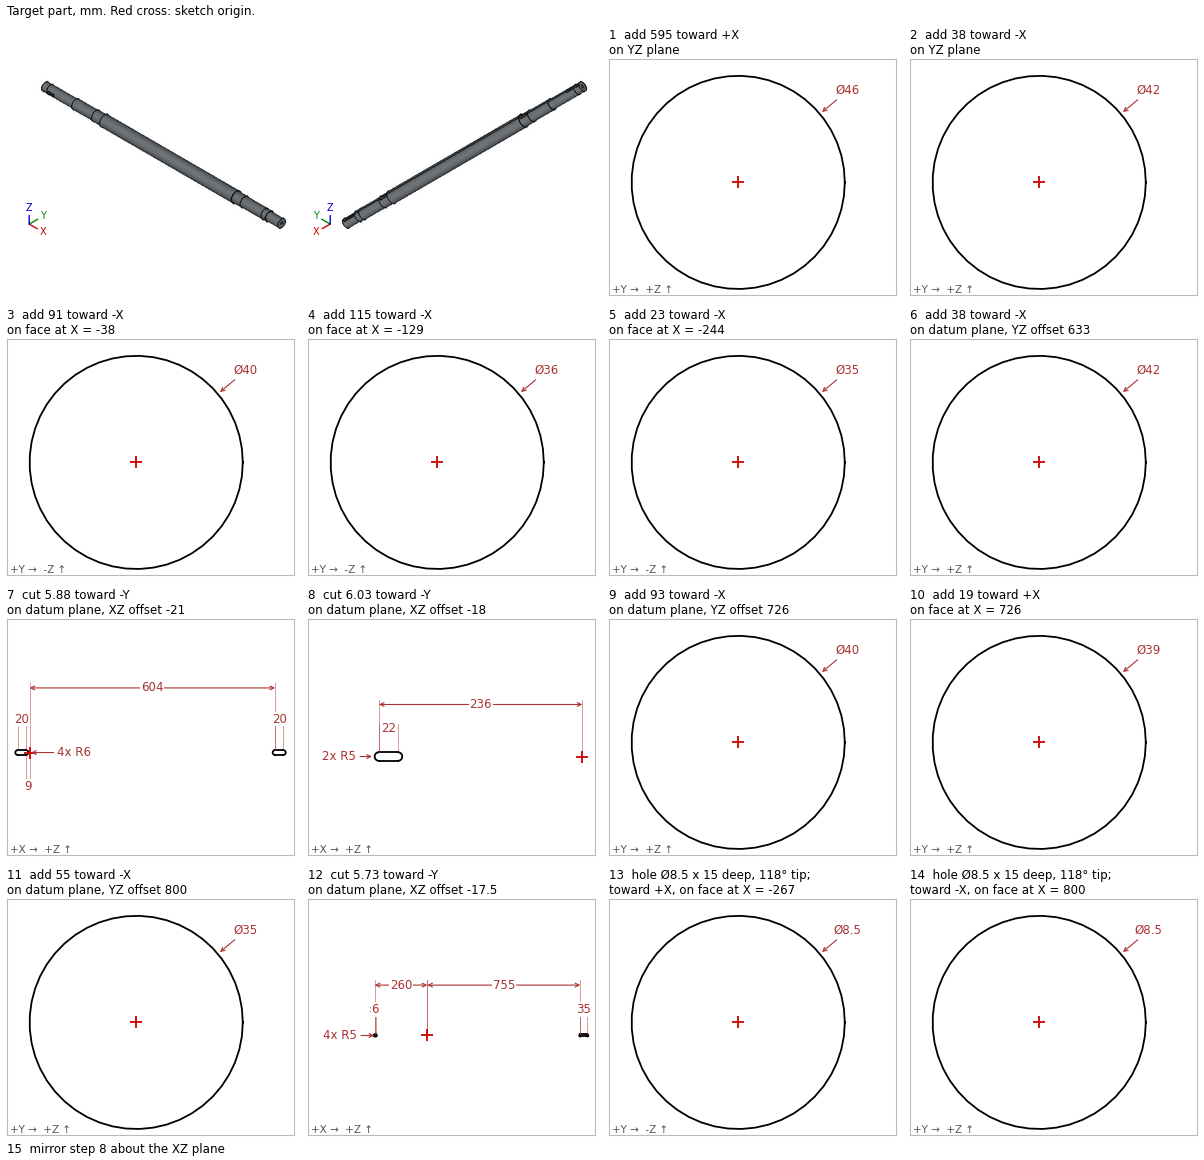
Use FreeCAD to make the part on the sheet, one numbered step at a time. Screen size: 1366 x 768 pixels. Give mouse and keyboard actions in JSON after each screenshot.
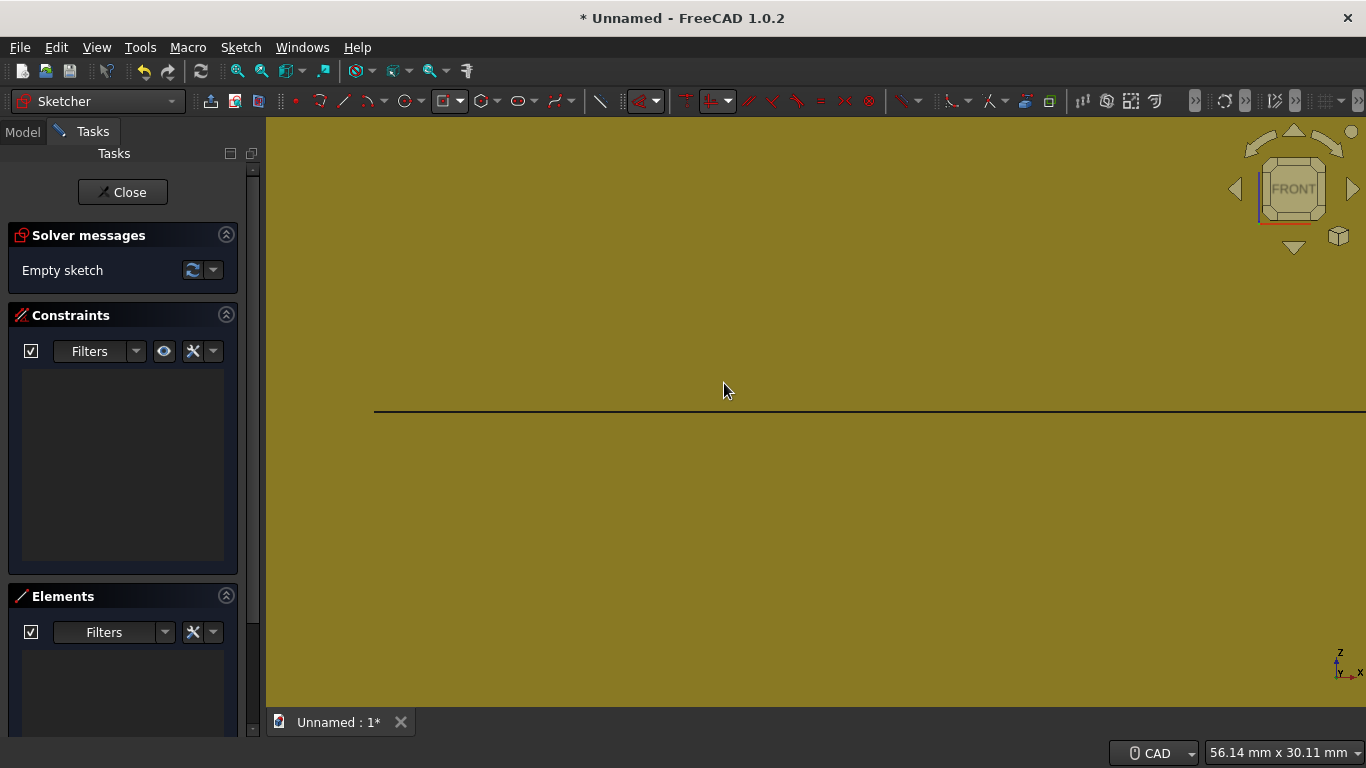
{"action": "key", "text": "g s"}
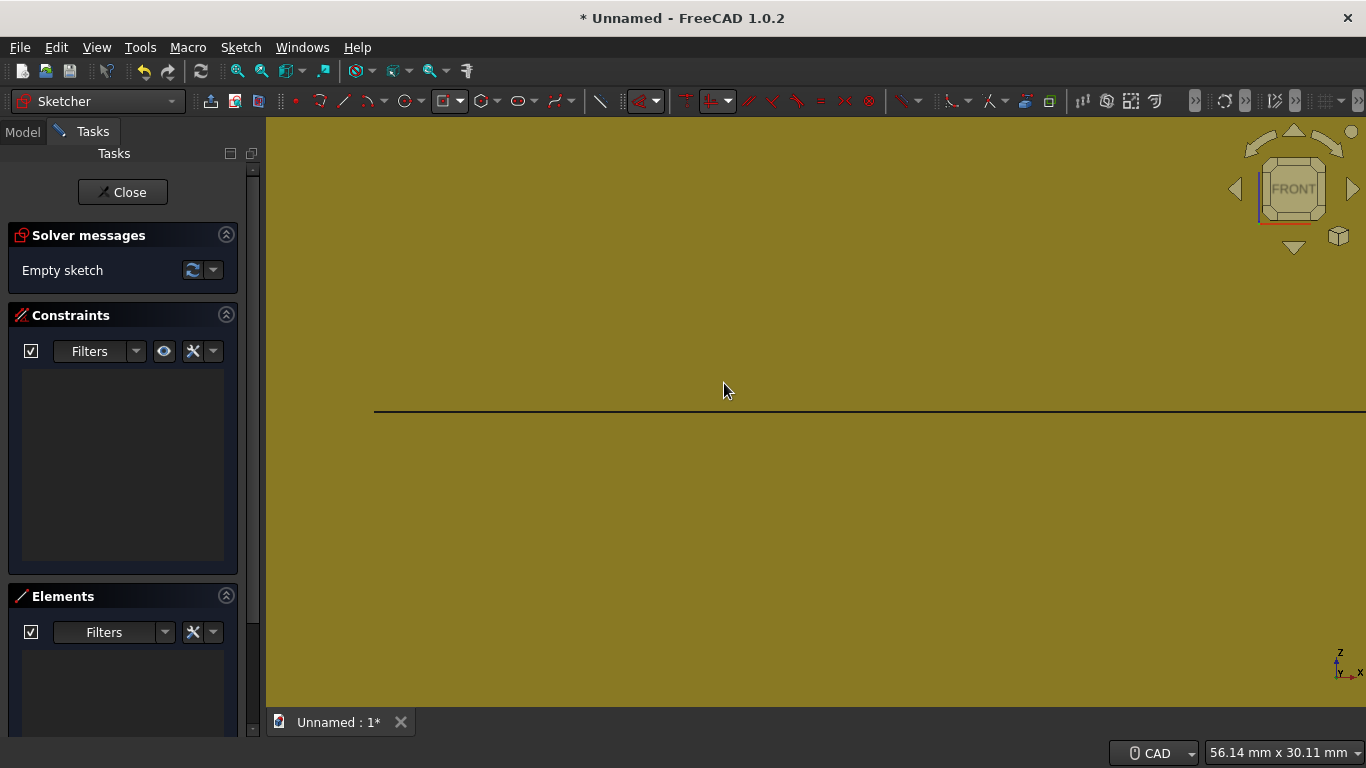
{"action": "left_click", "coordinate": [532, 412]}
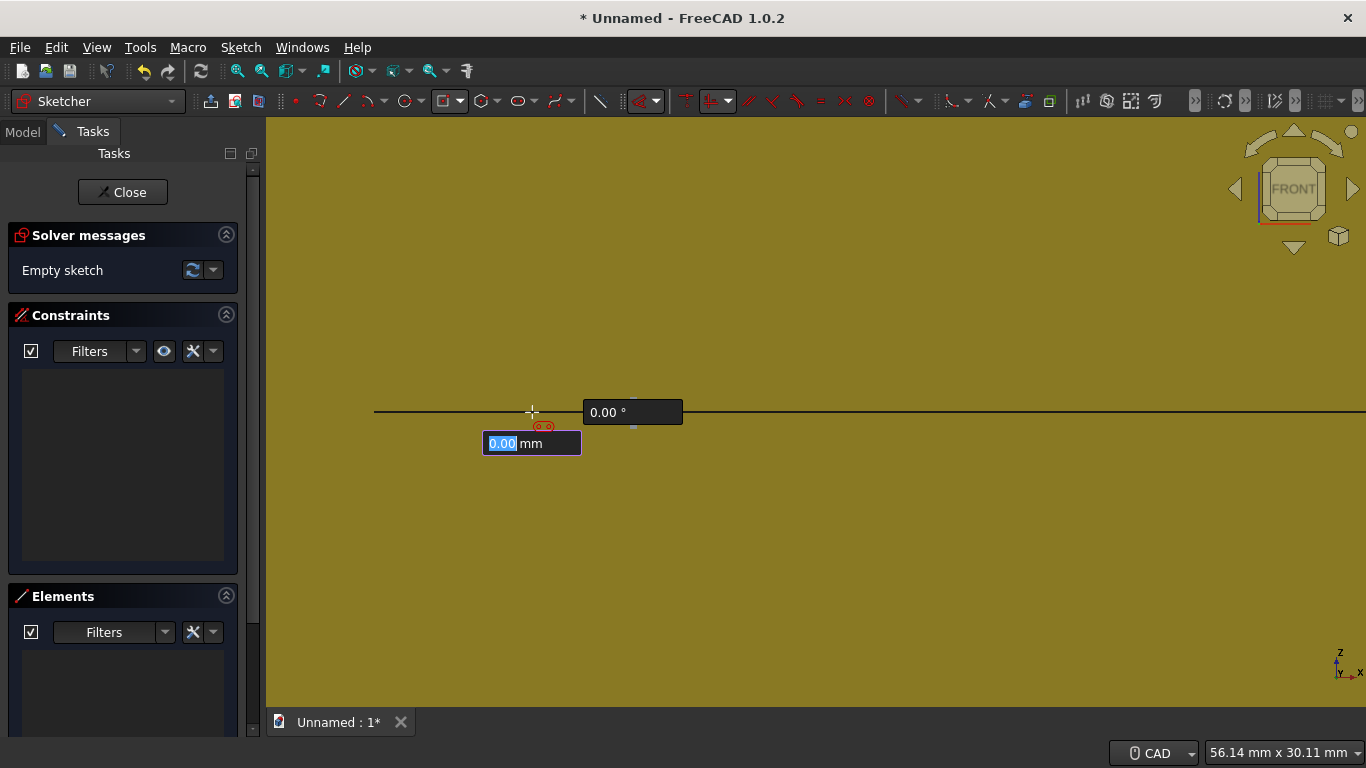
{"action": "left_click", "coordinate": [963, 403]}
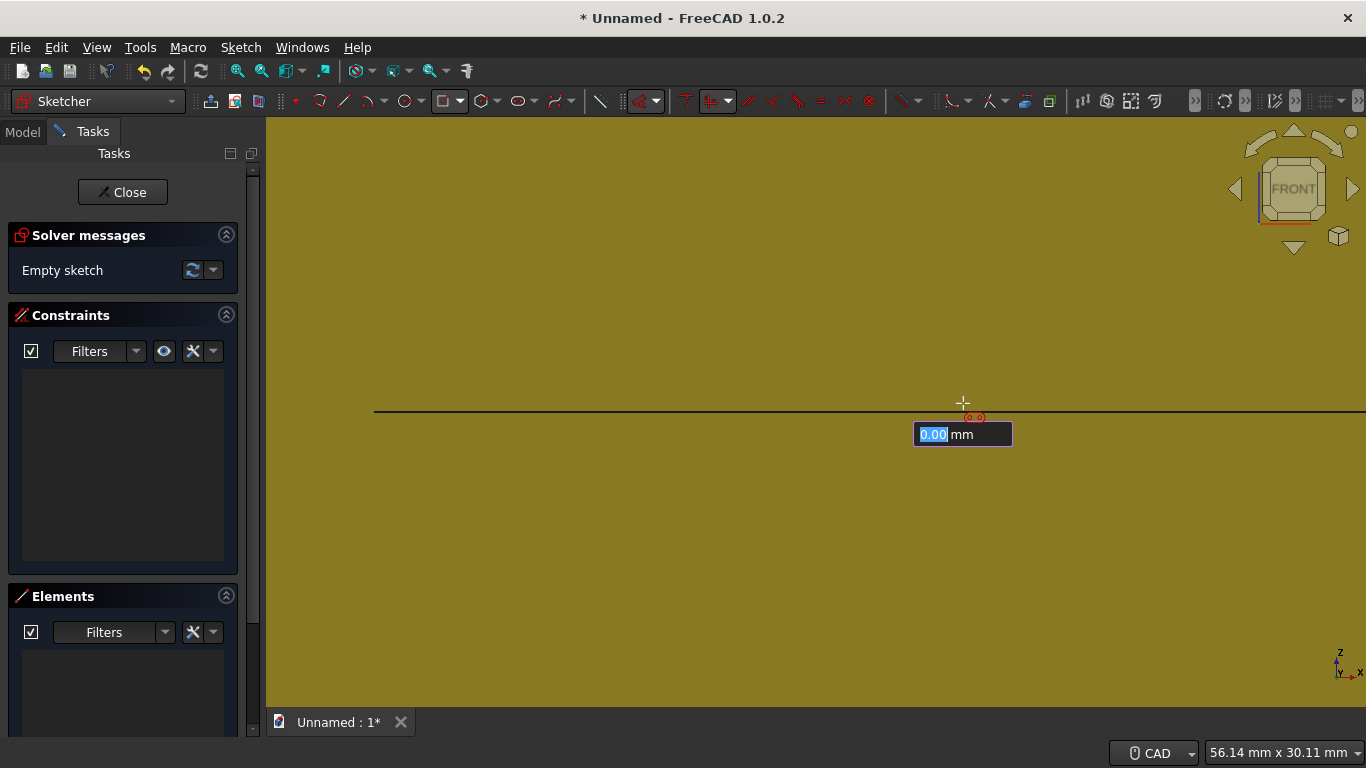
{"action": "left_click", "coordinate": [747, 510]}
{"action": "key", "text": "Escape"}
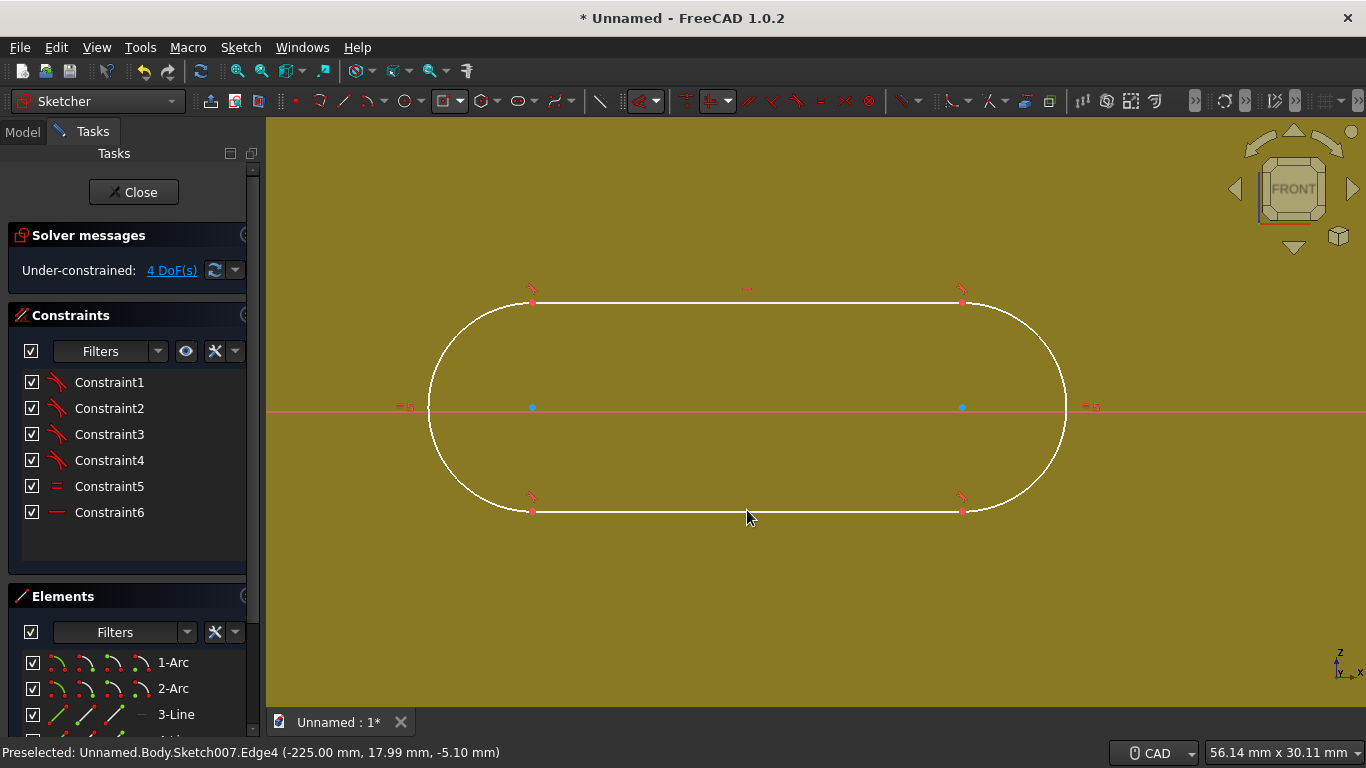
{"action": "left_click", "coordinate": [533, 407]}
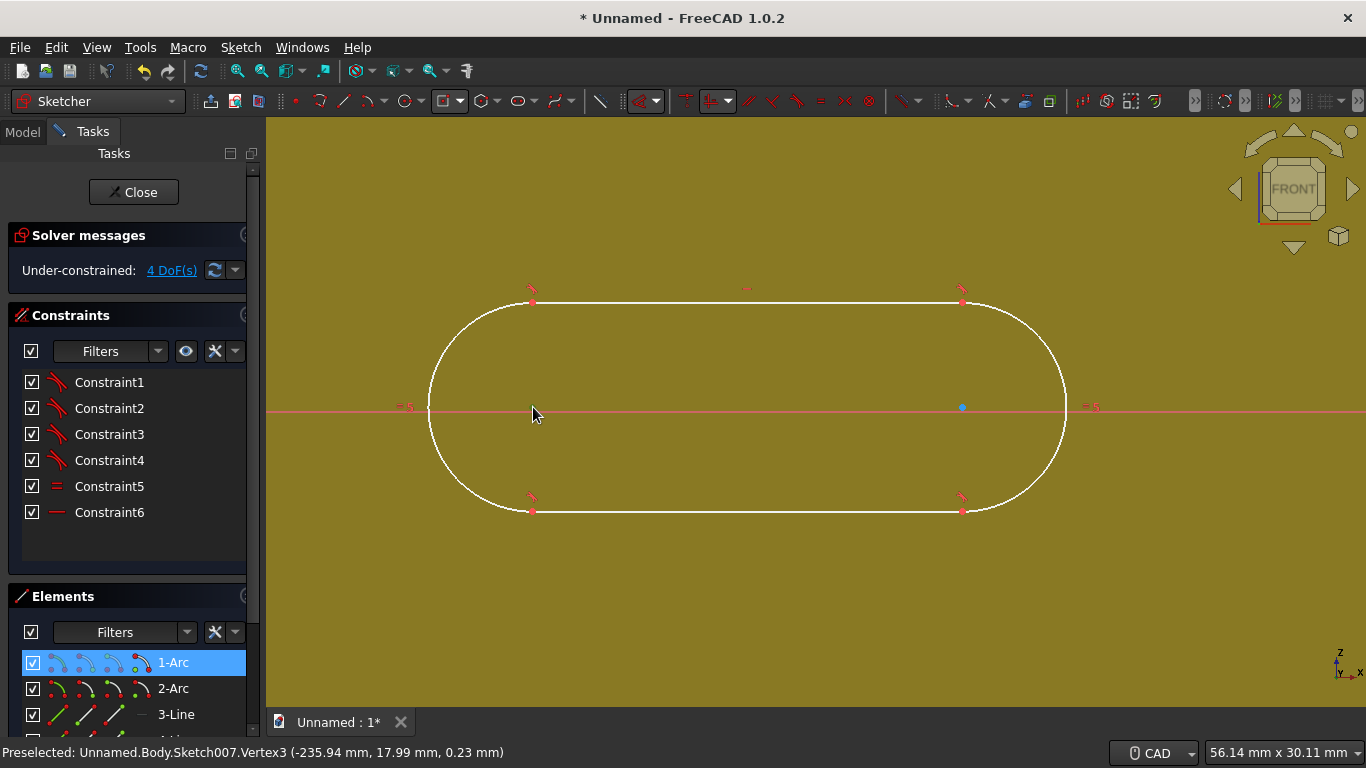
{"action": "left_click", "coordinate": [359, 412]}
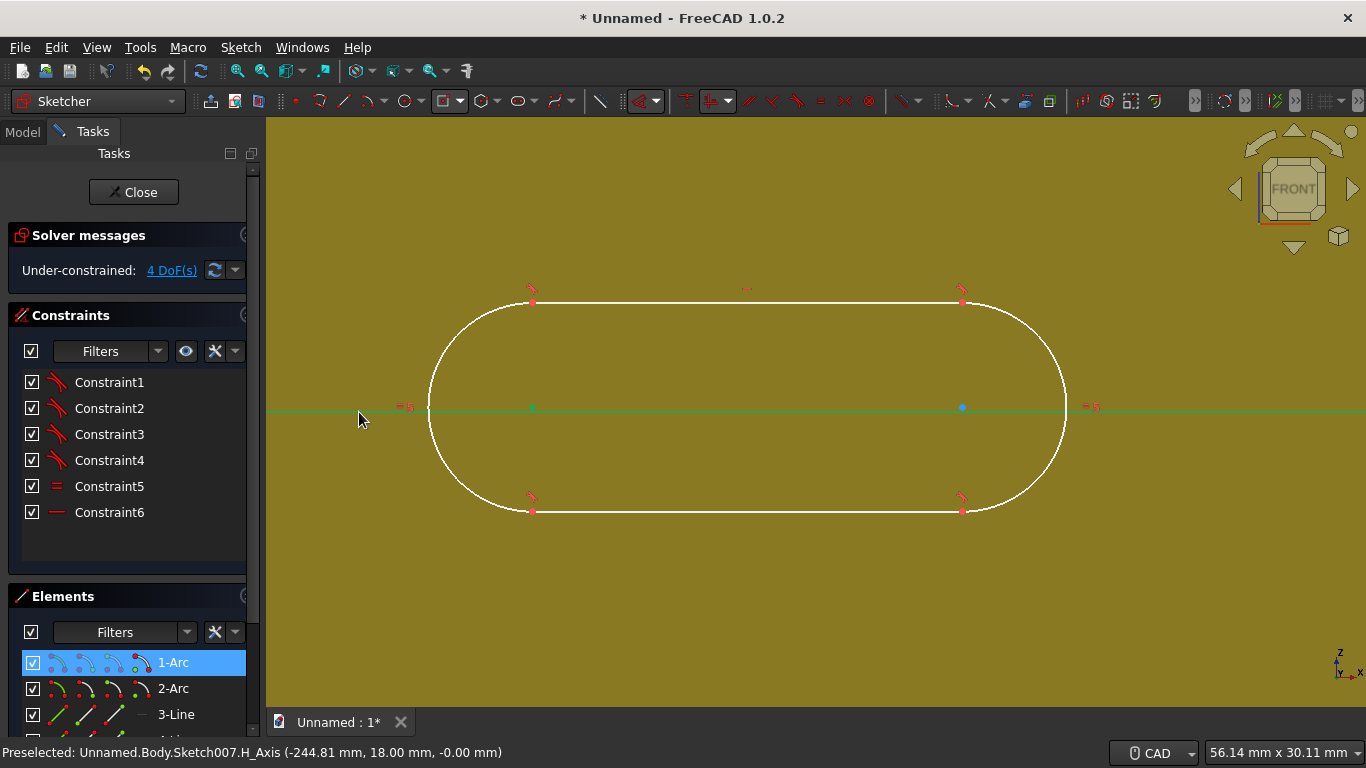
{"action": "key", "text": "c"}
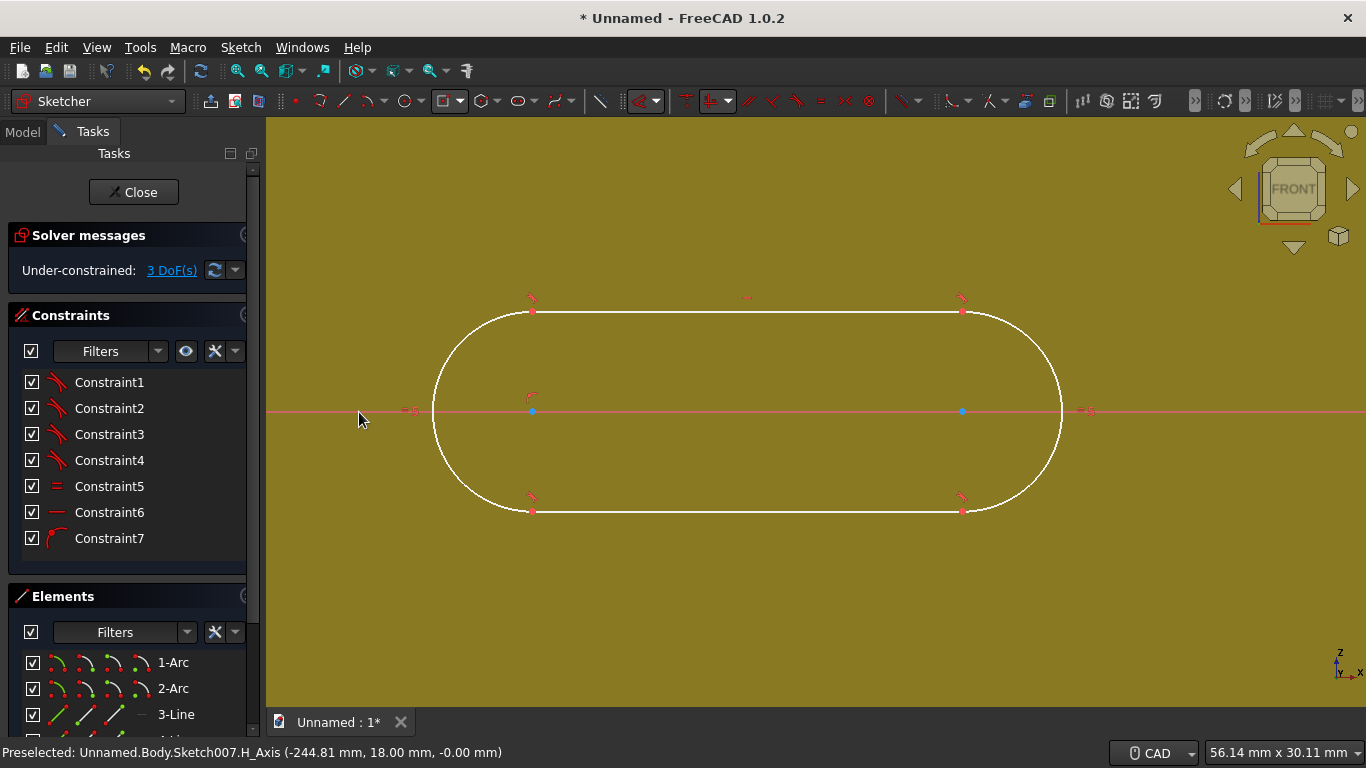
{"action": "left_click", "coordinate": [452, 353]}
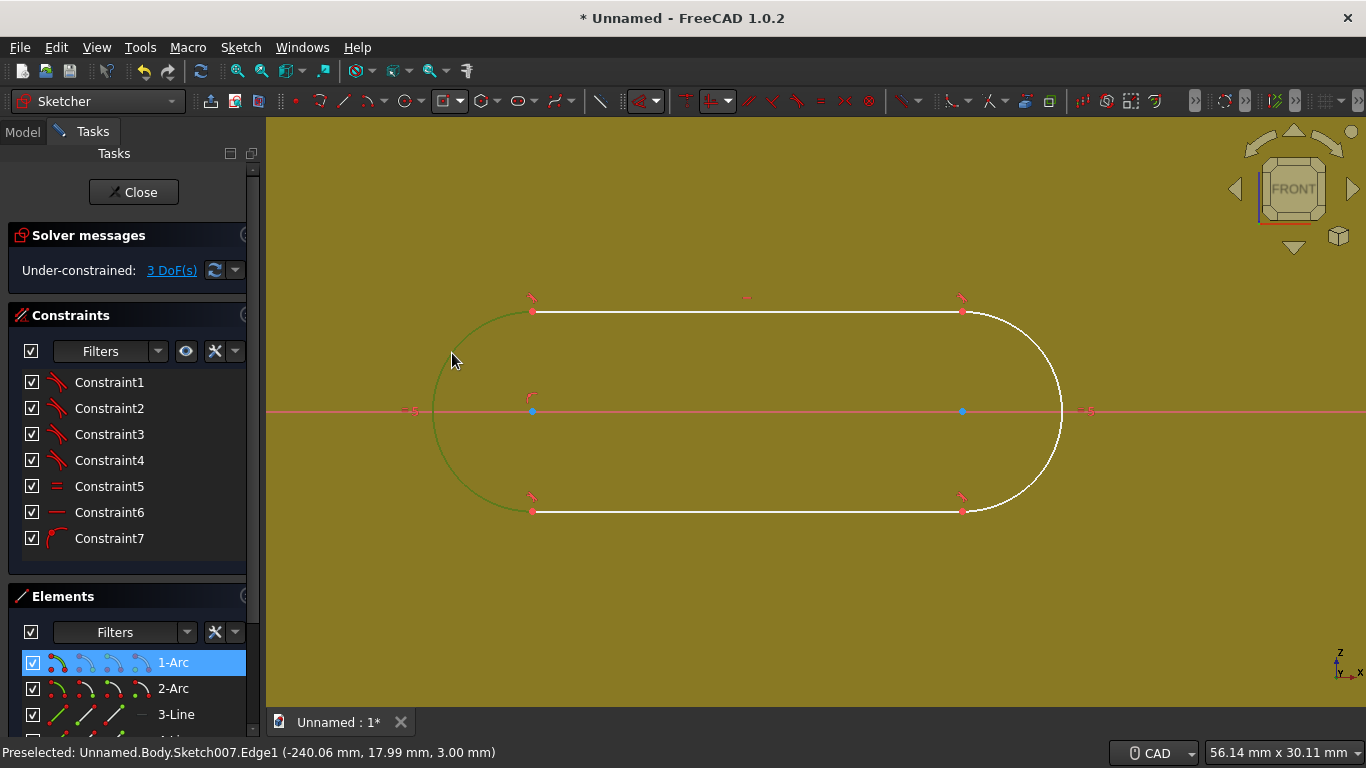
{"action": "key", "text": "k r"}